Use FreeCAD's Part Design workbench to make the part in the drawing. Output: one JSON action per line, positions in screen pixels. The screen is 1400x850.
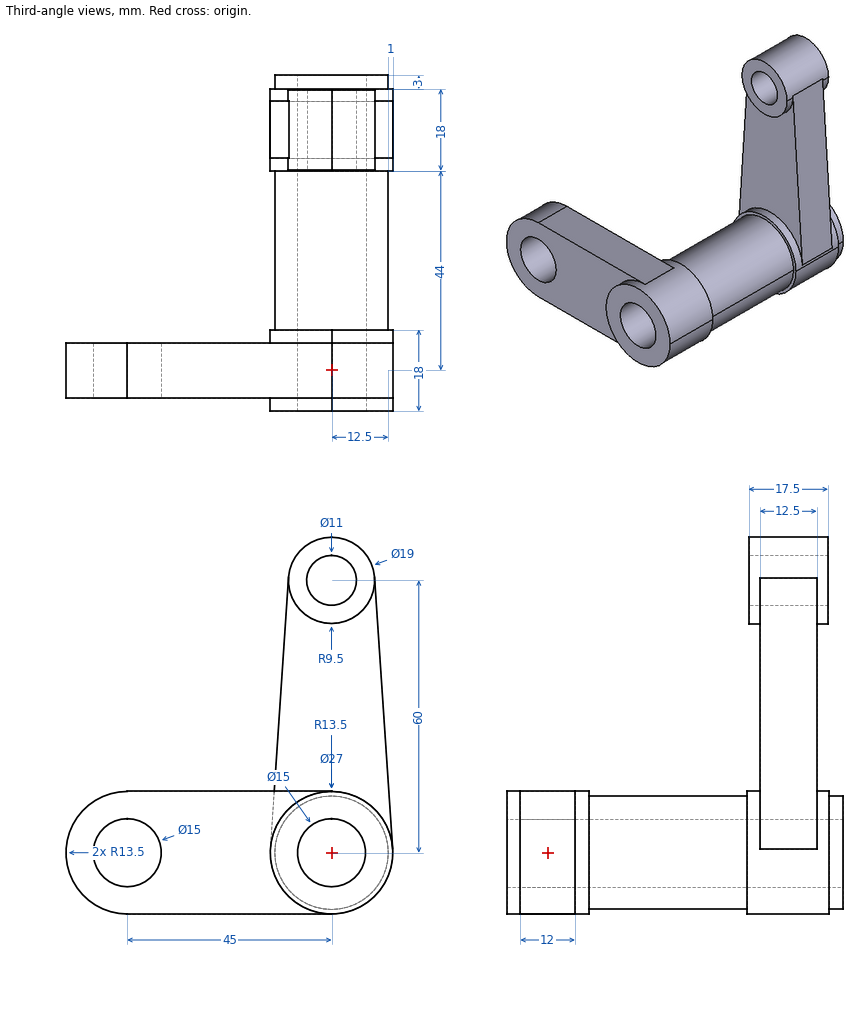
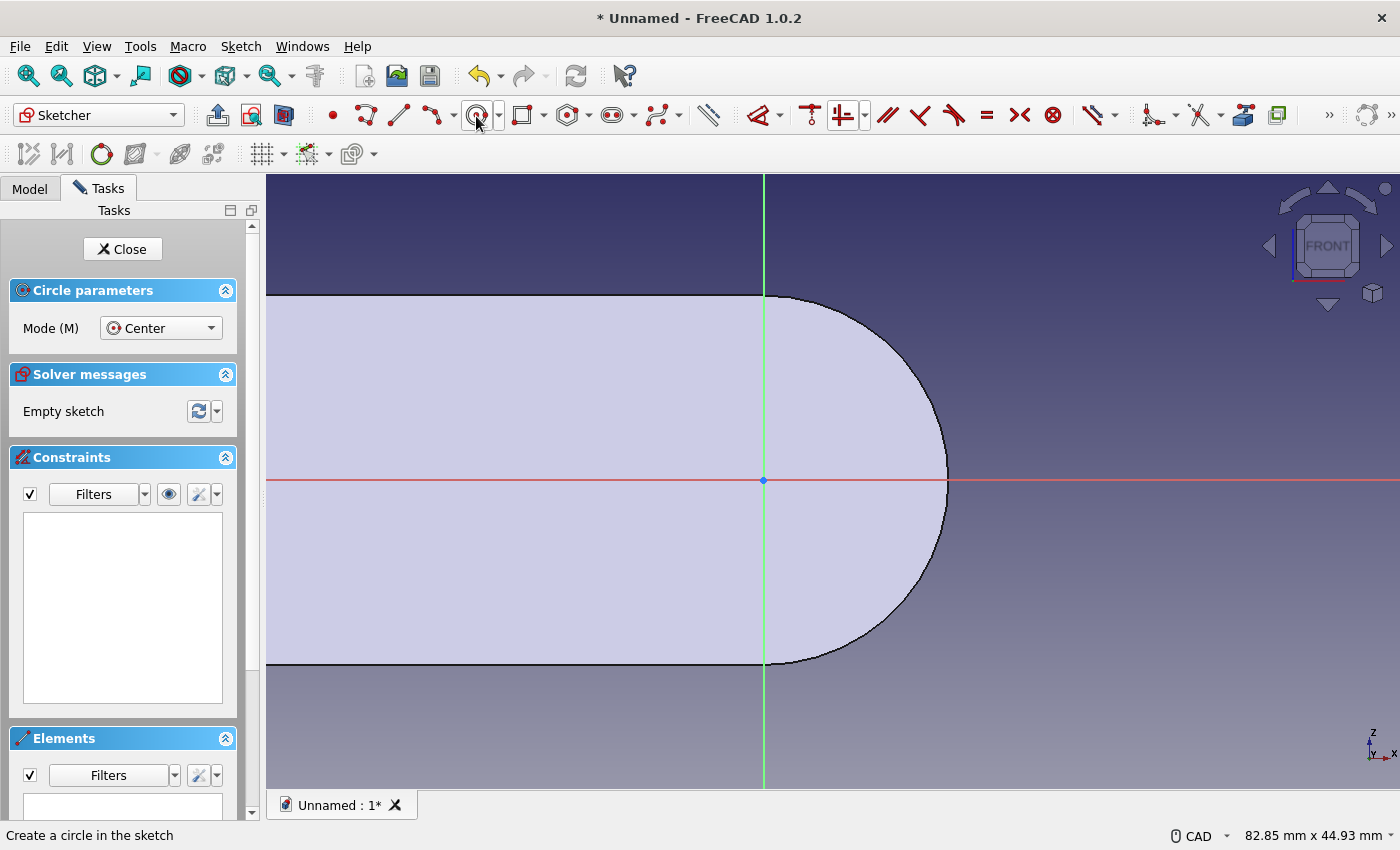
{"action": "left_click", "coordinate": [764, 480]}
{"action": "left_click", "coordinate": [894, 350]}
{"action": "key", "text": "Escape"}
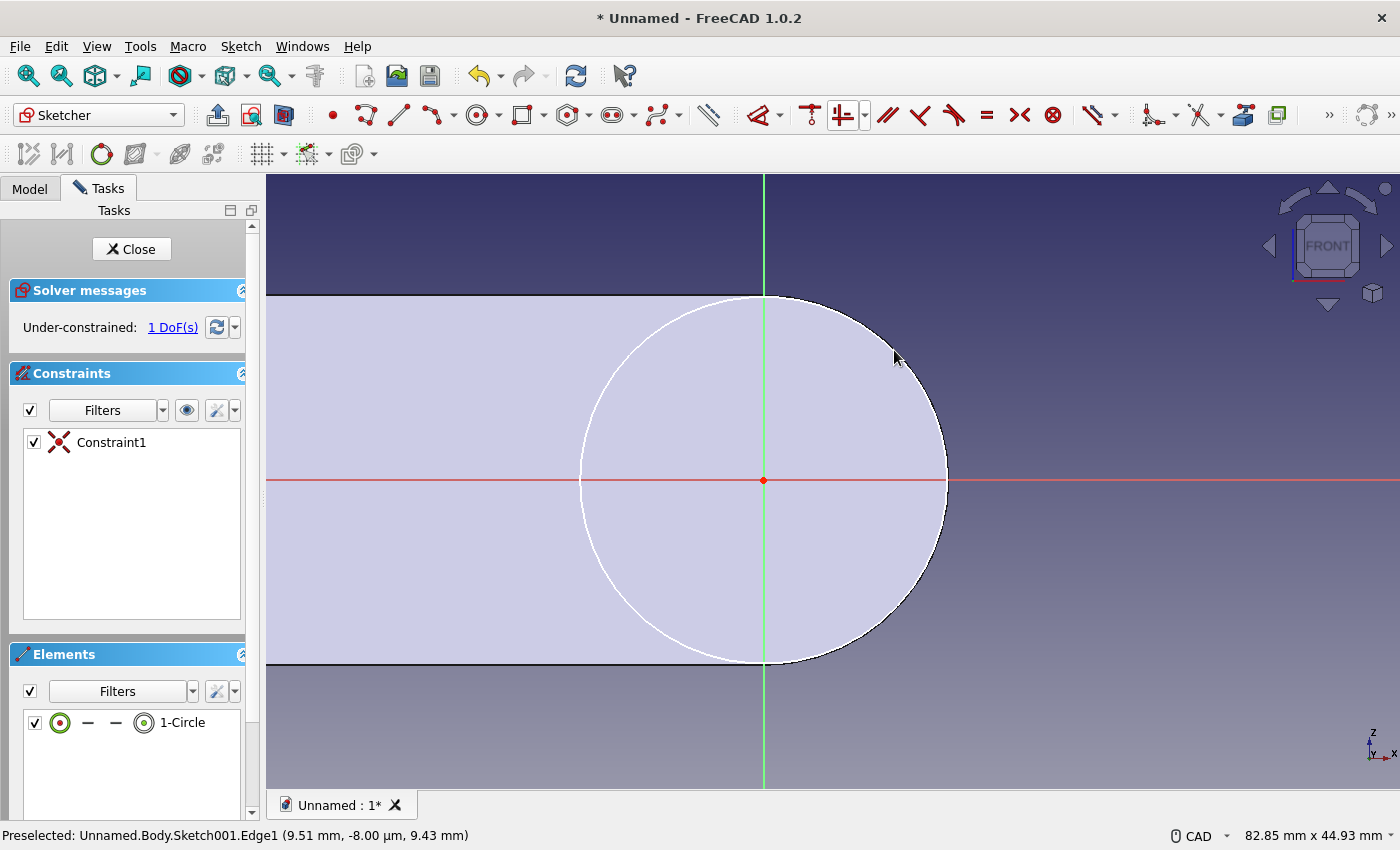
{"action": "key", "text": "d"}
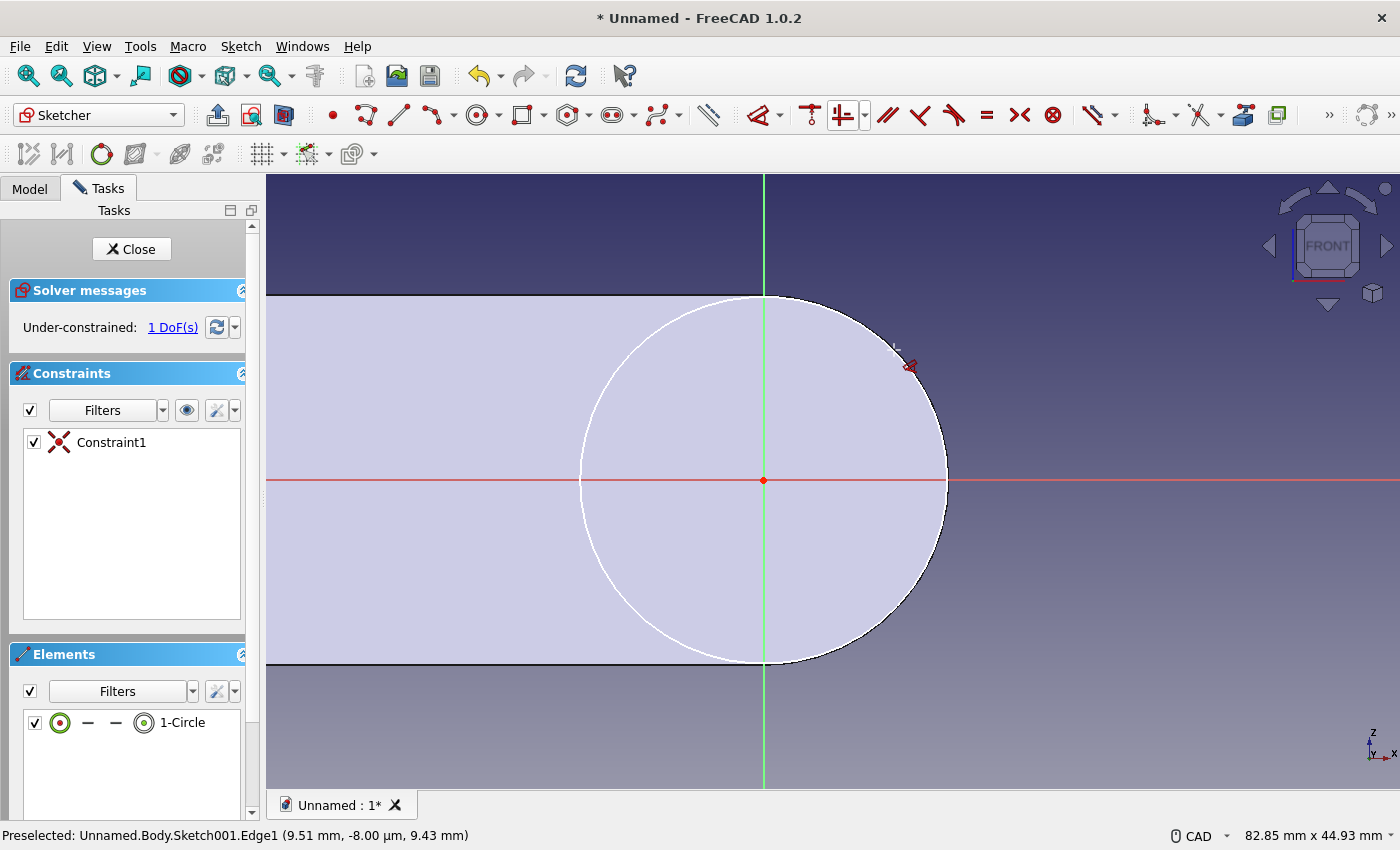
{"action": "left_click", "coordinate": [893, 350]}
{"action": "left_click", "coordinate": [916, 327]}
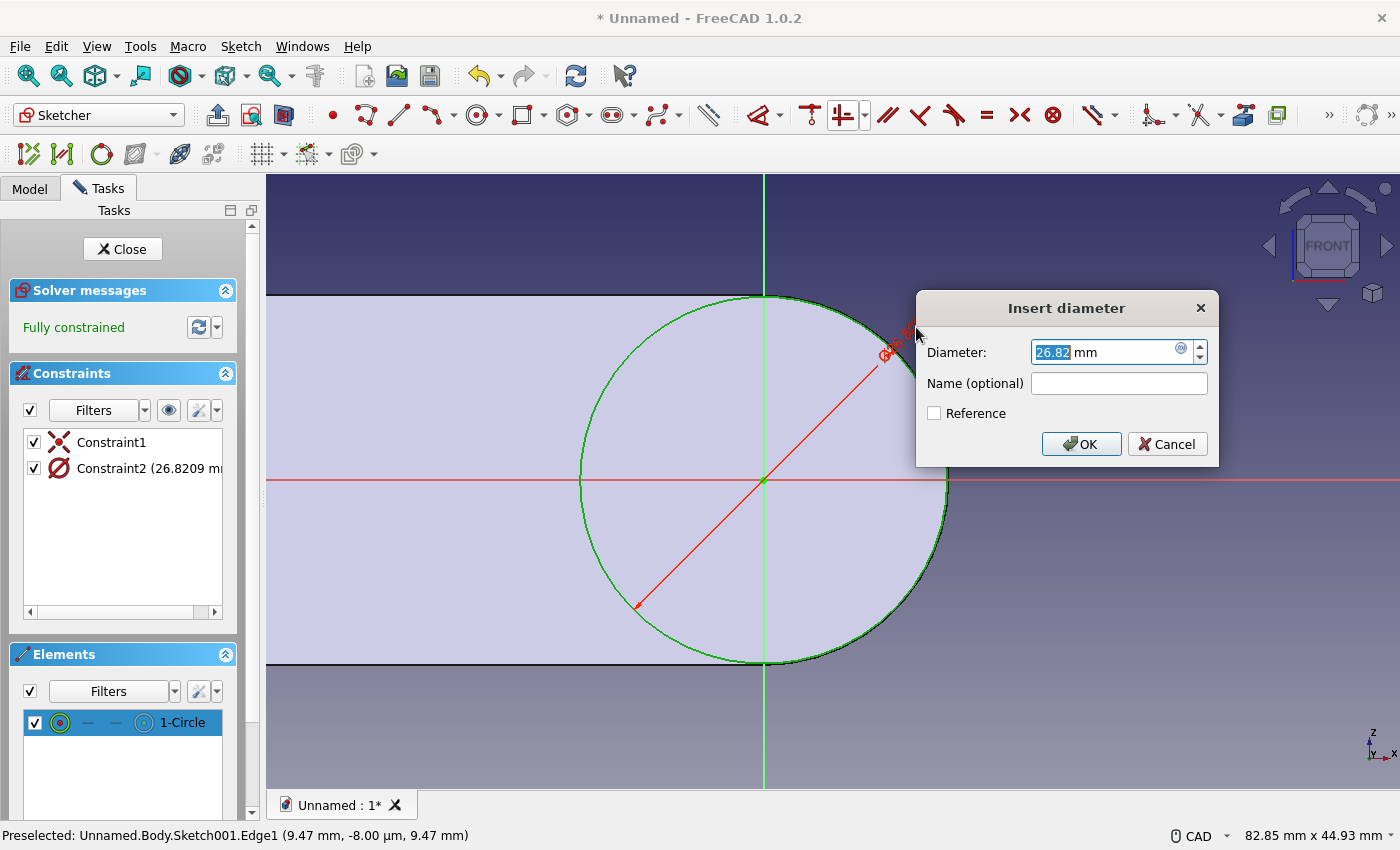
{"action": "type", "text": "27"}
{"action": "key", "text": "Return"}
{"action": "key", "text": "Escape"}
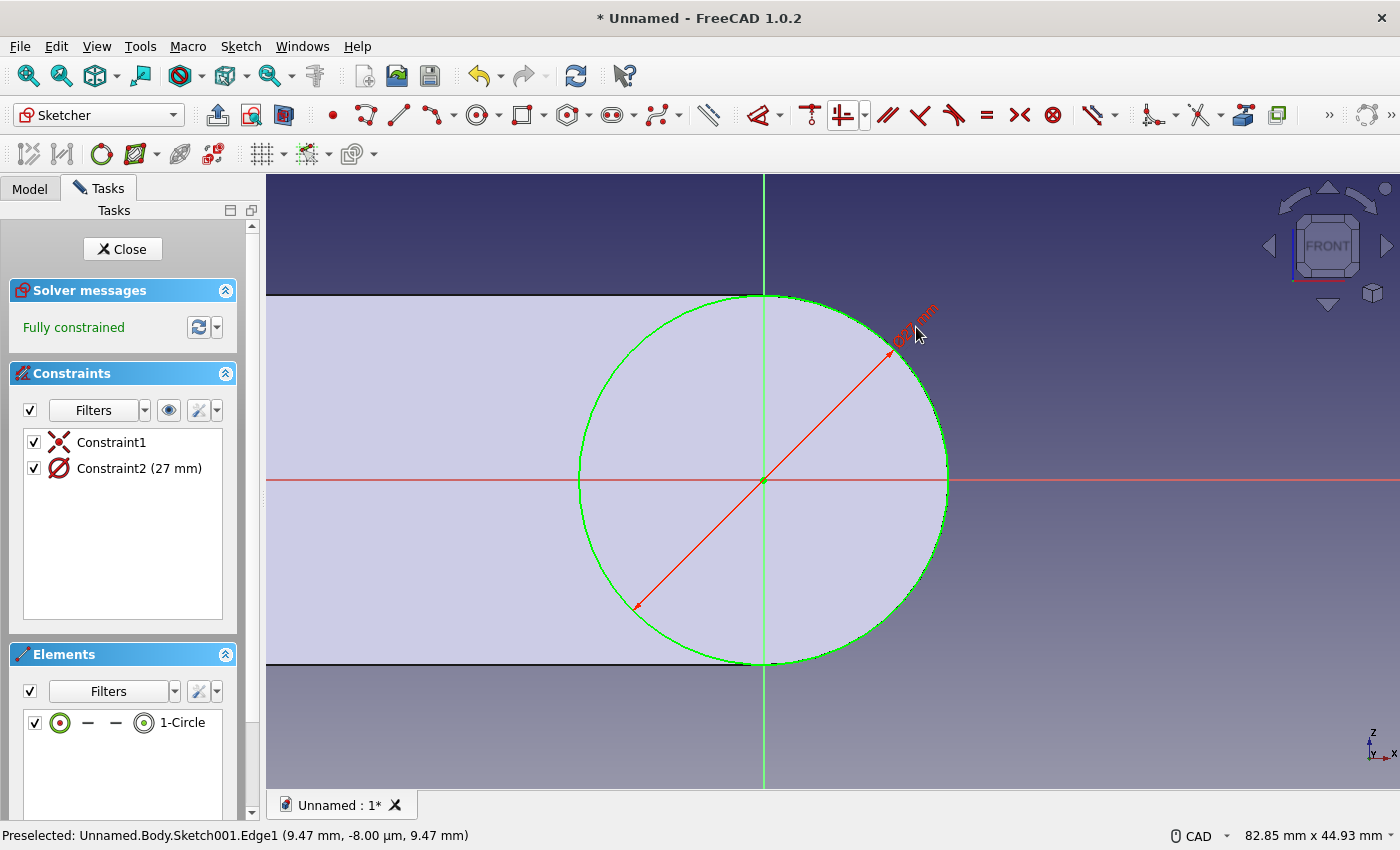
{"action": "left_click", "coordinate": [123, 249]}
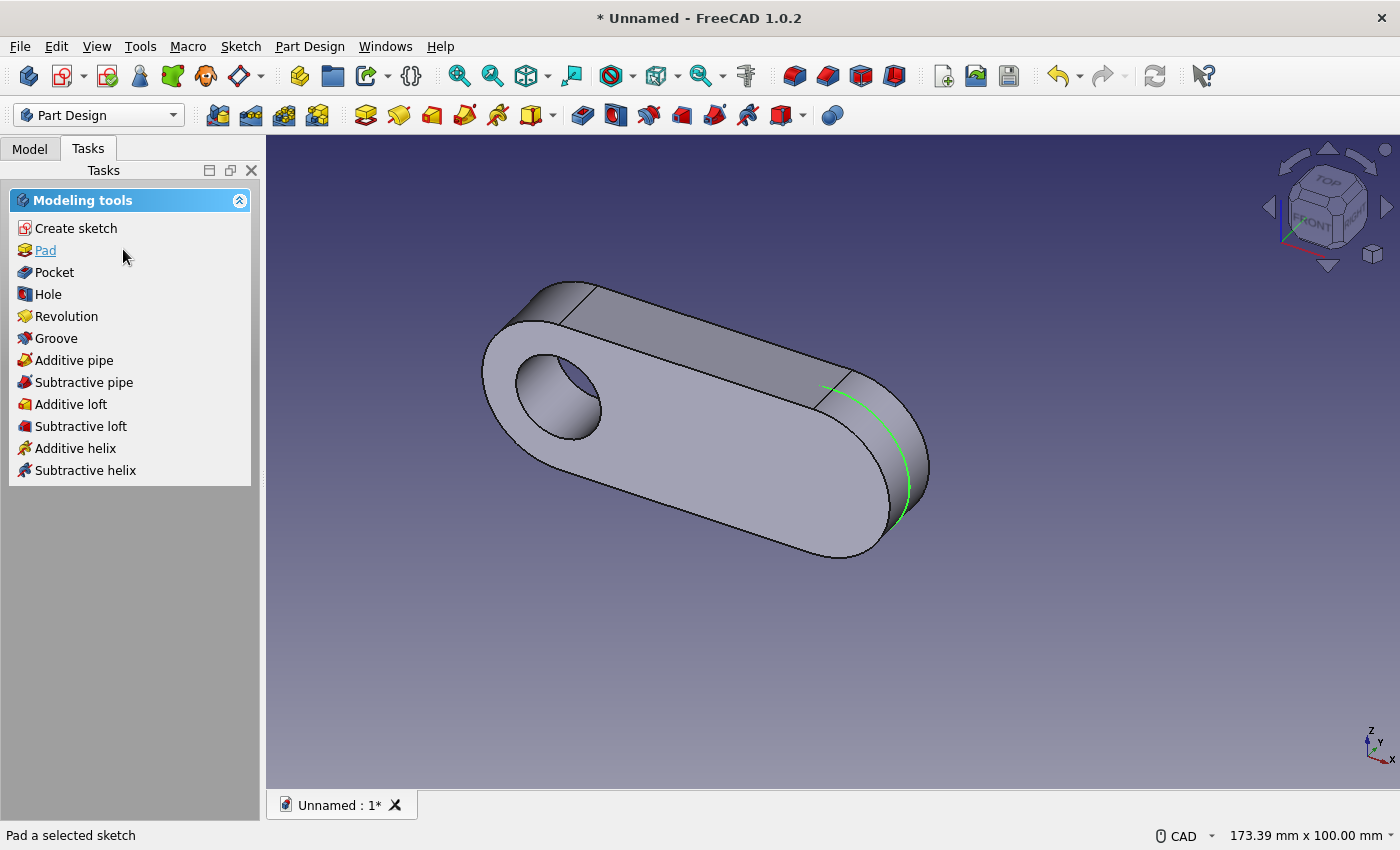
{"action": "left_click", "coordinate": [366, 116]}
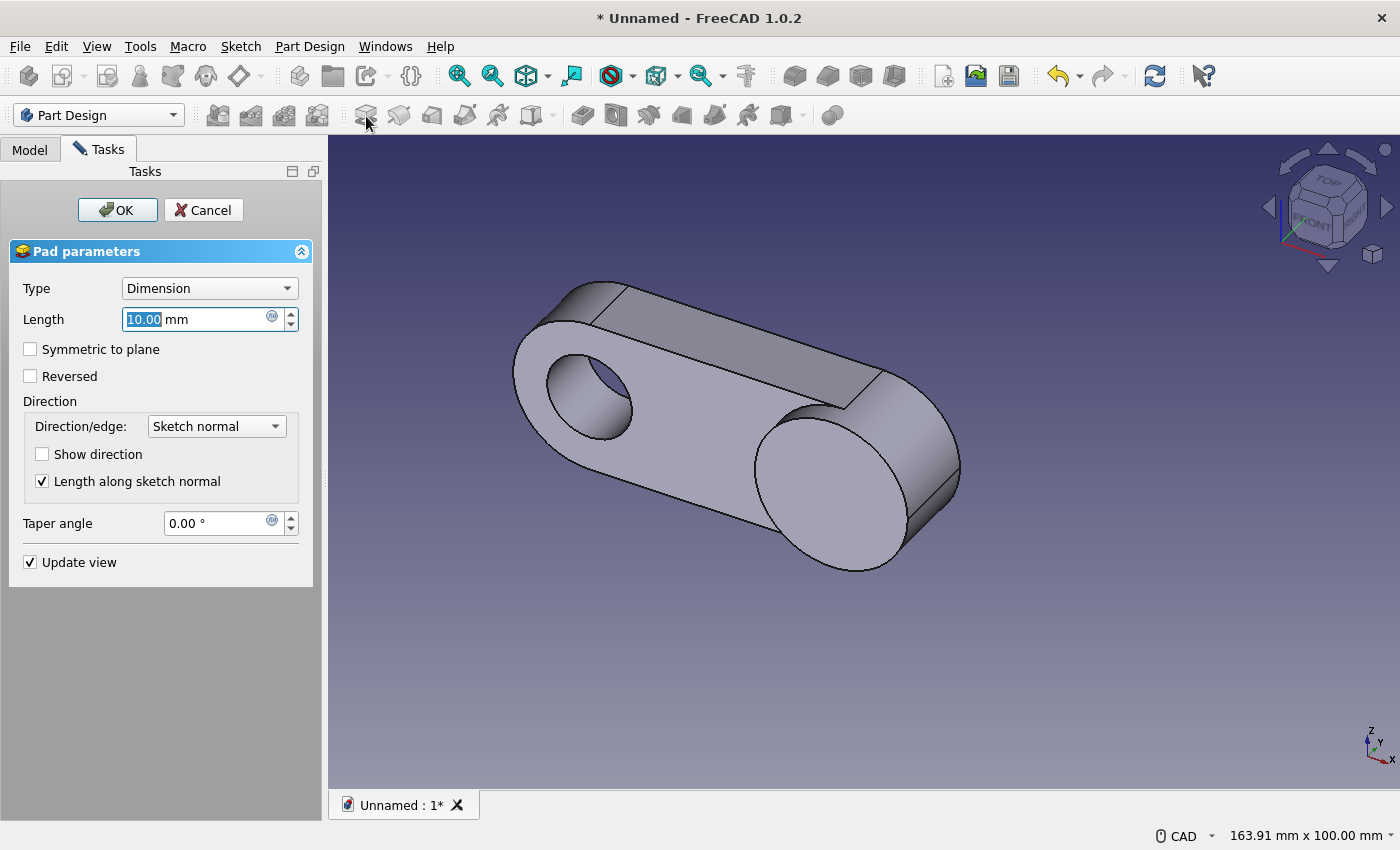
{"action": "type", "text": "18"}
{"action": "key", "text": "Tab"}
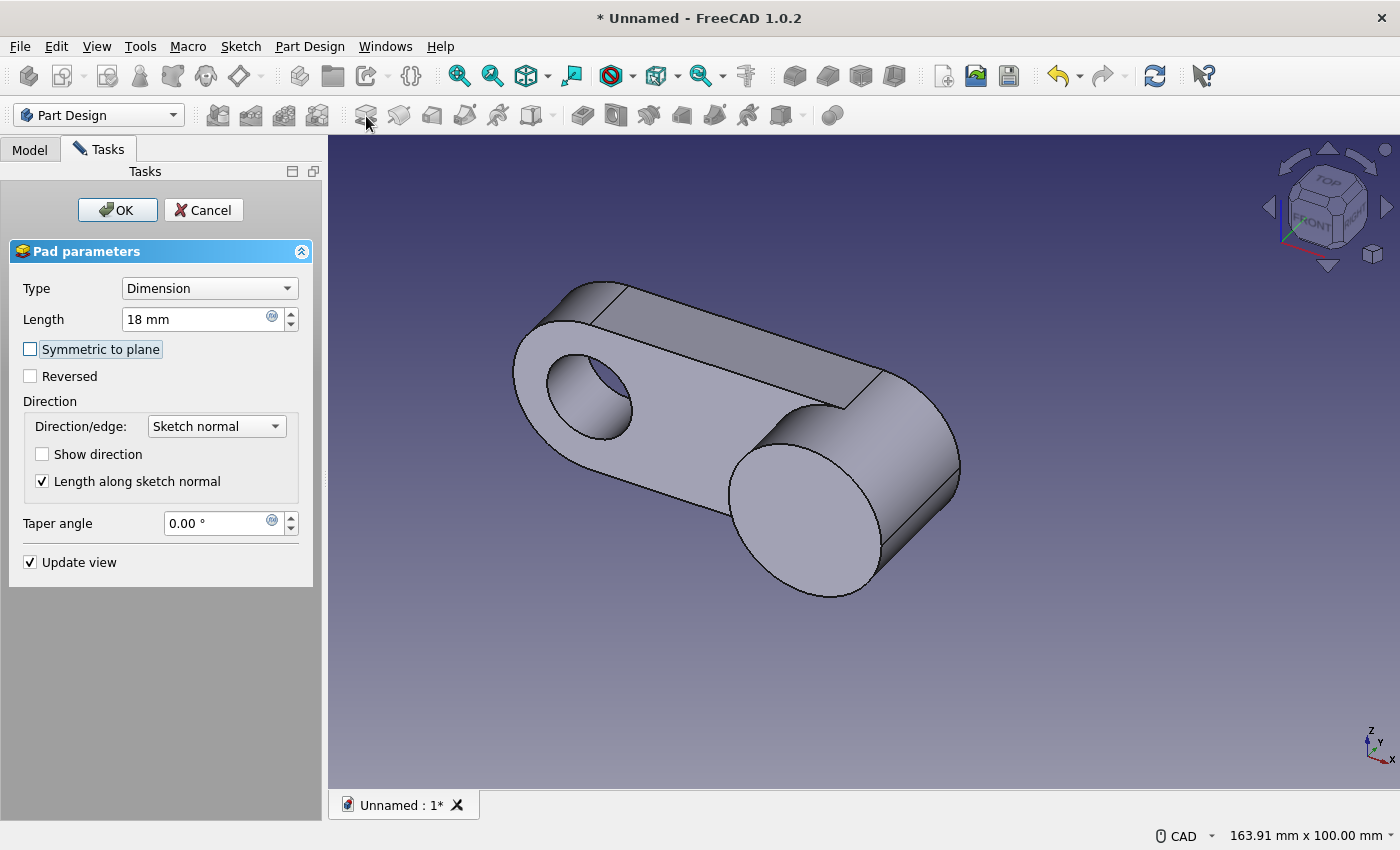
{"action": "left_click", "coordinate": [31, 349]}